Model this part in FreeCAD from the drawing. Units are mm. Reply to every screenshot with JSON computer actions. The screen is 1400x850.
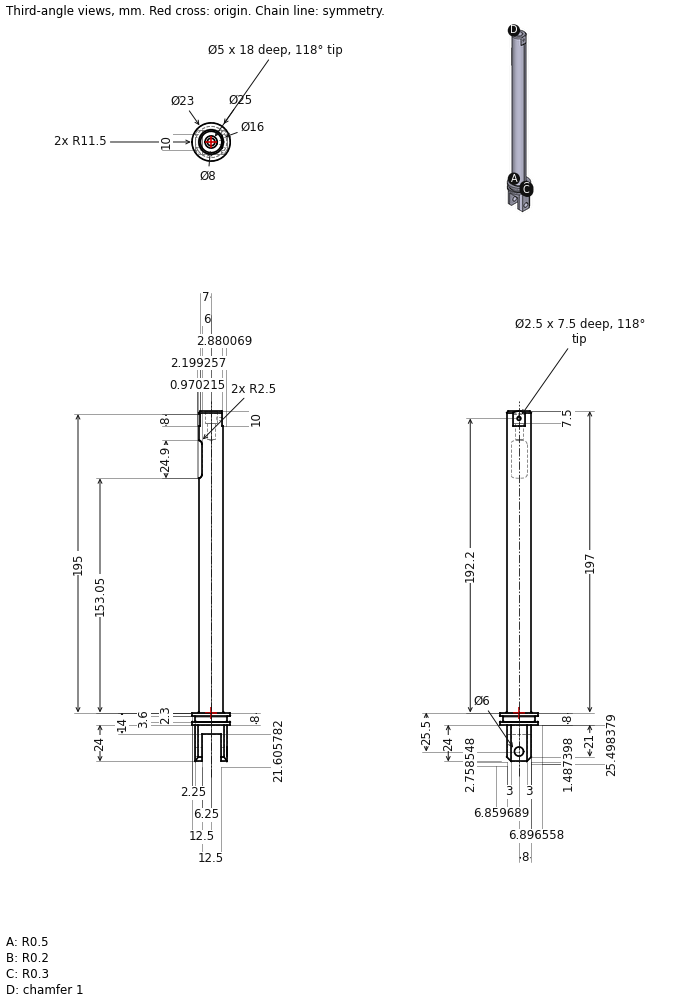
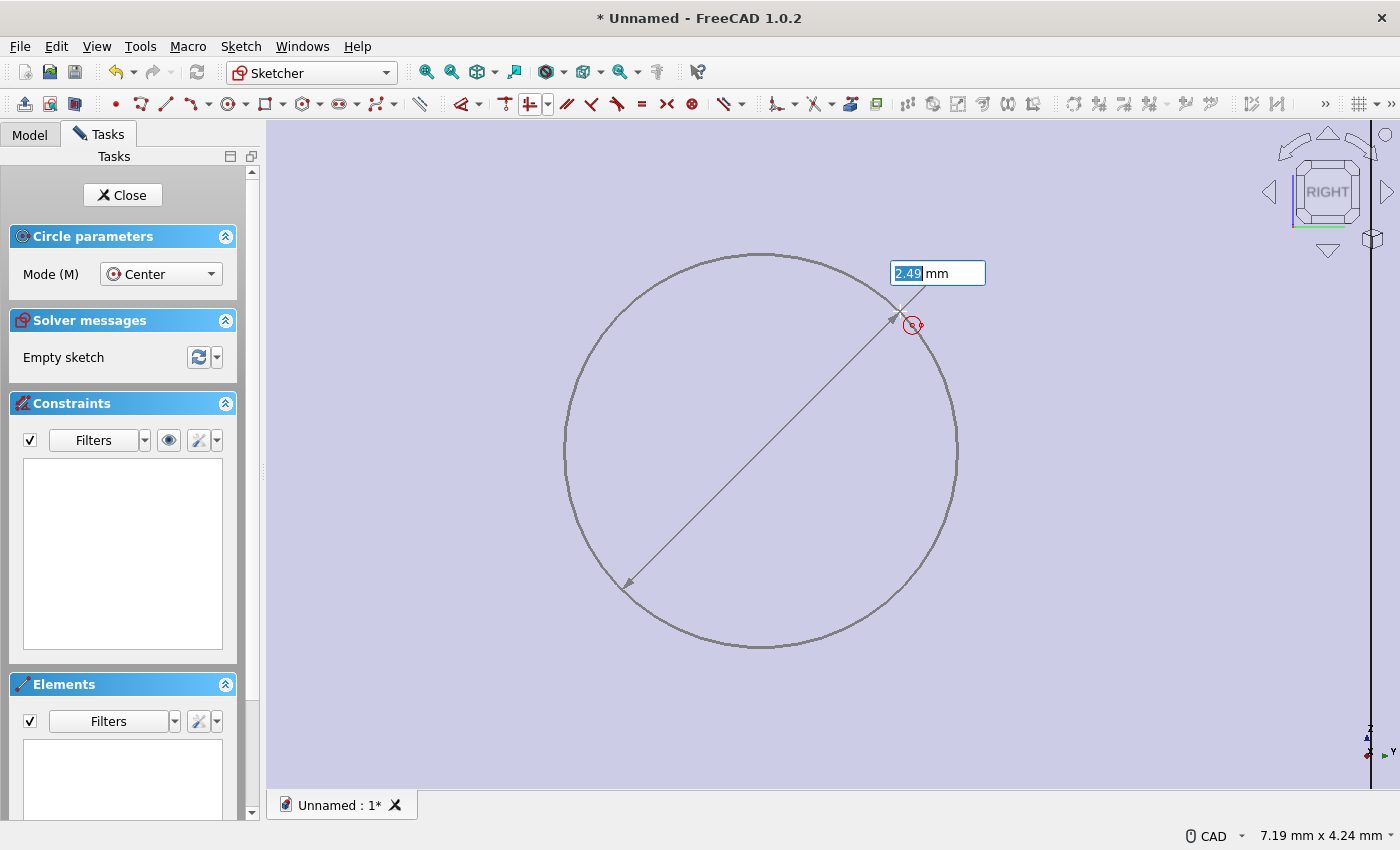
{"action": "type", "text": "2.5"}
{"action": "key", "text": "Return"}
{"action": "key", "text": "Escape"}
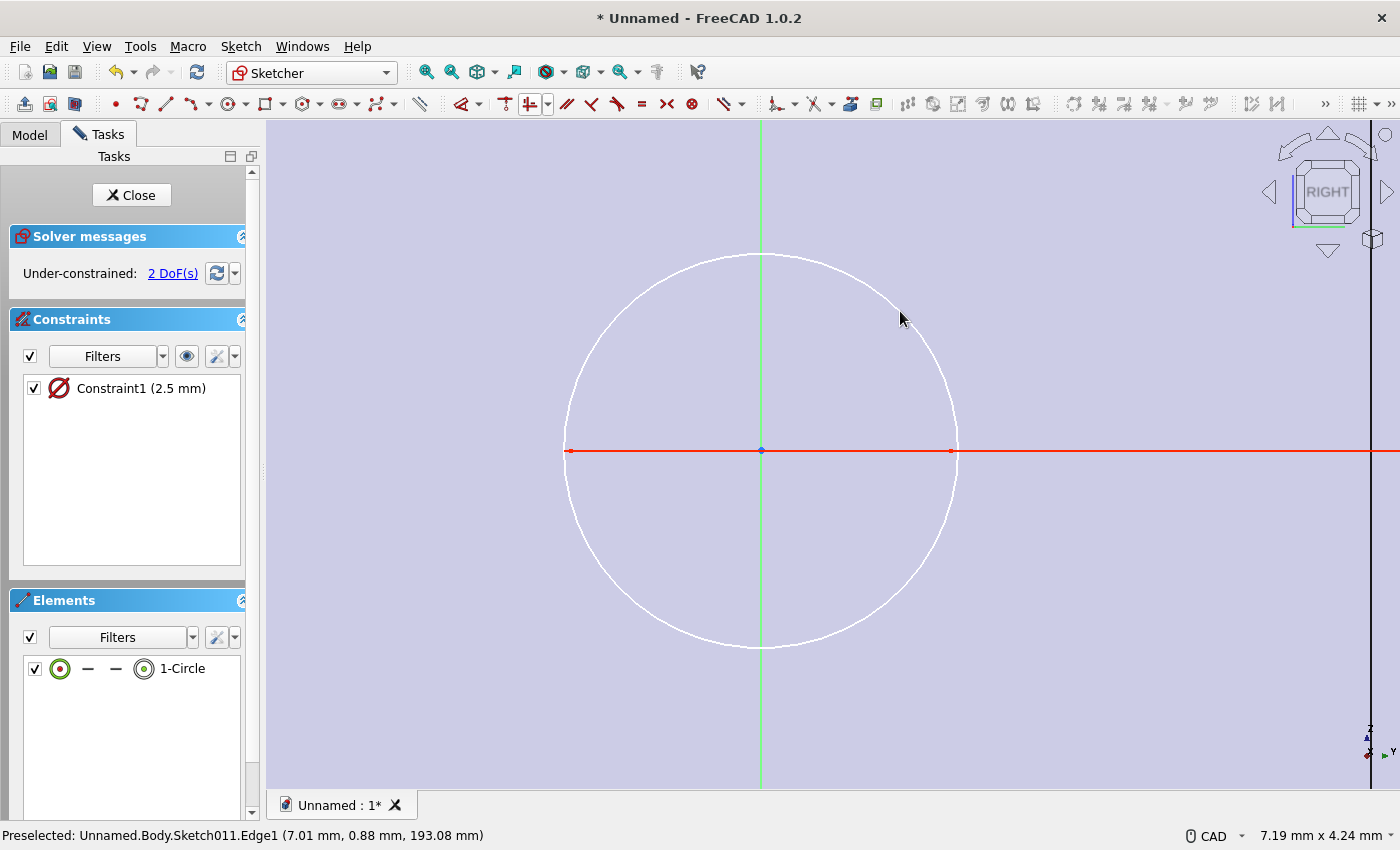
{"action": "left_click", "coordinate": [761, 451]}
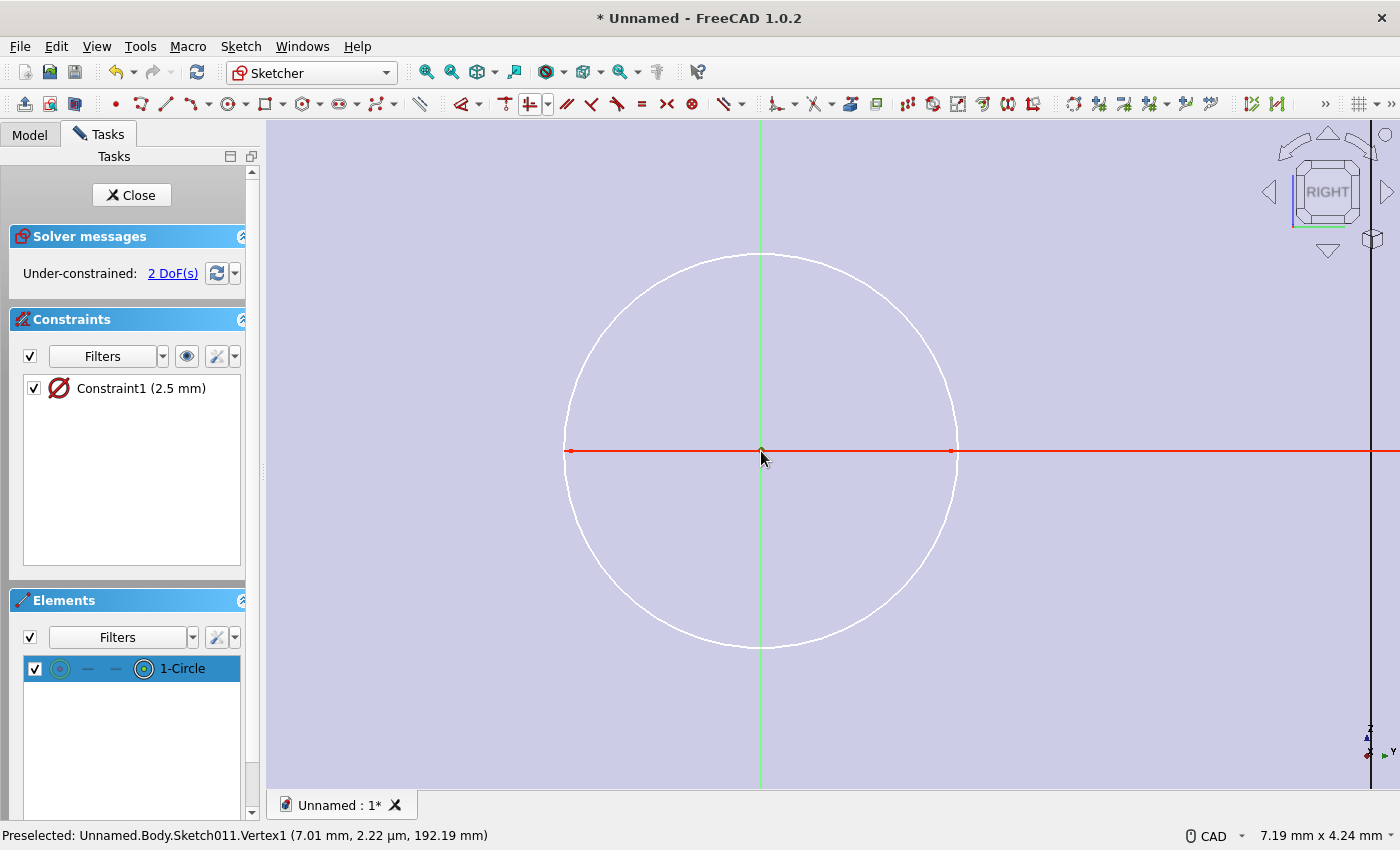
{"action": "left_click", "coordinate": [761, 717]}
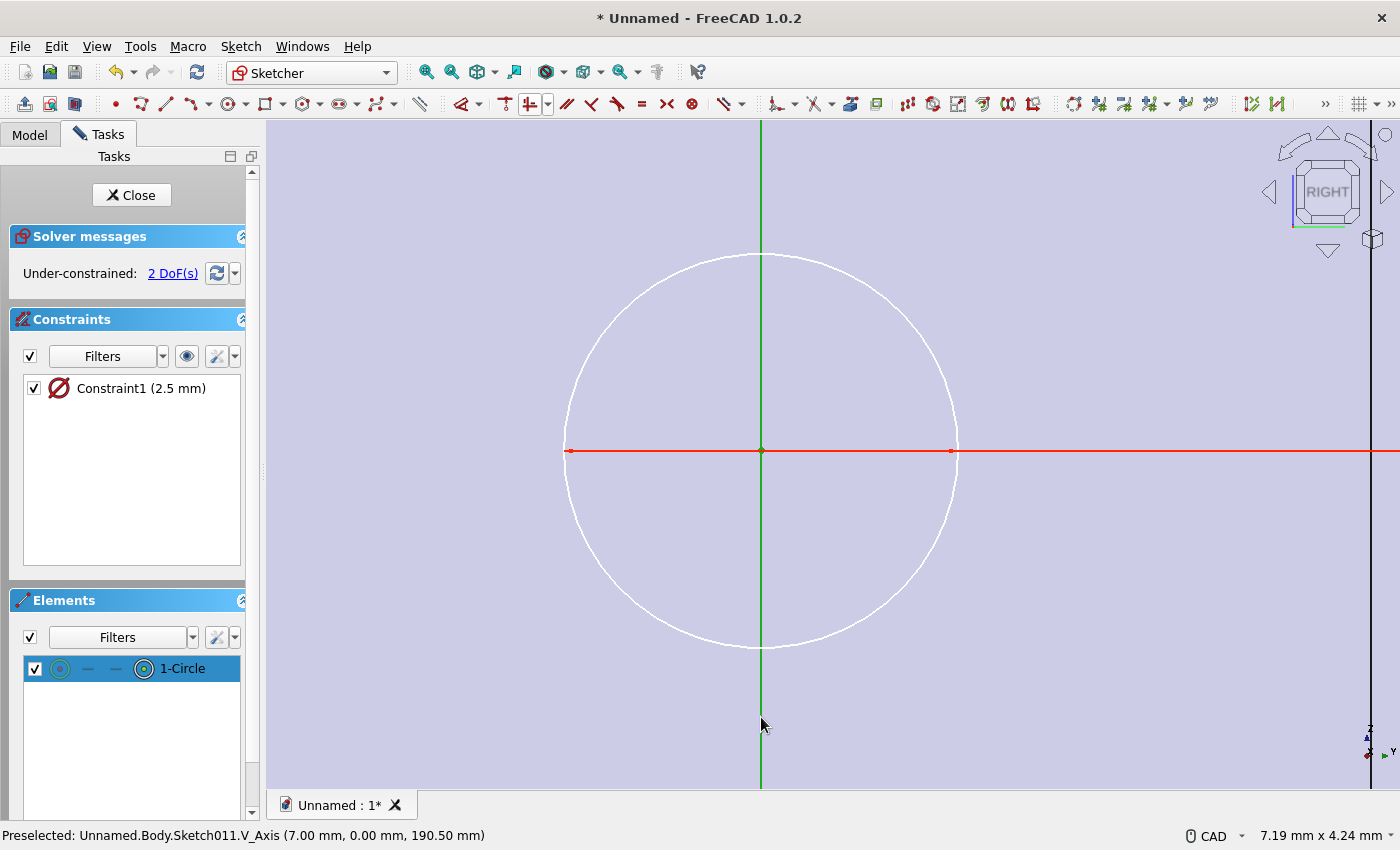
{"action": "left_click", "coordinate": [505, 104]}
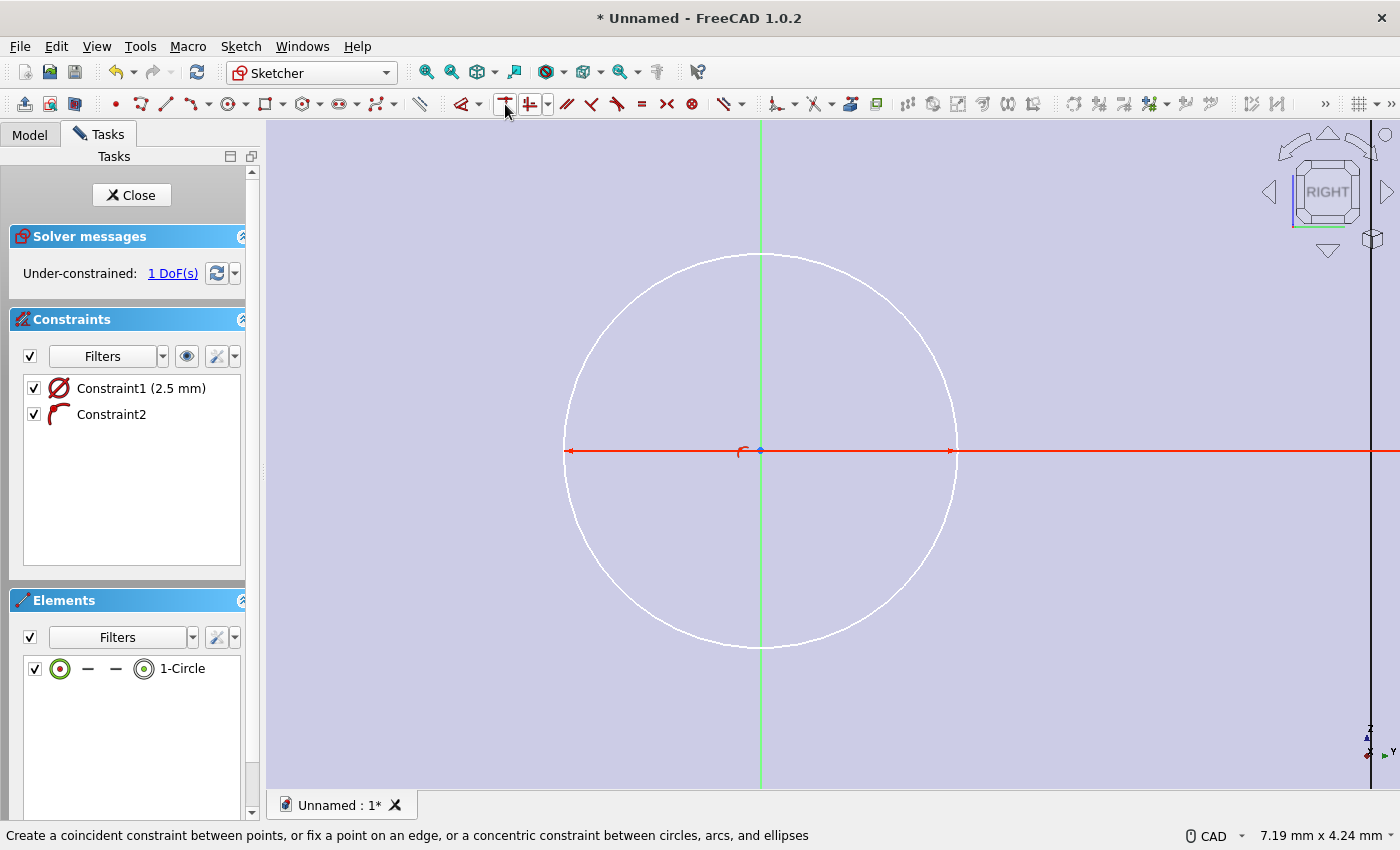
{"action": "left_click", "coordinate": [460, 104]}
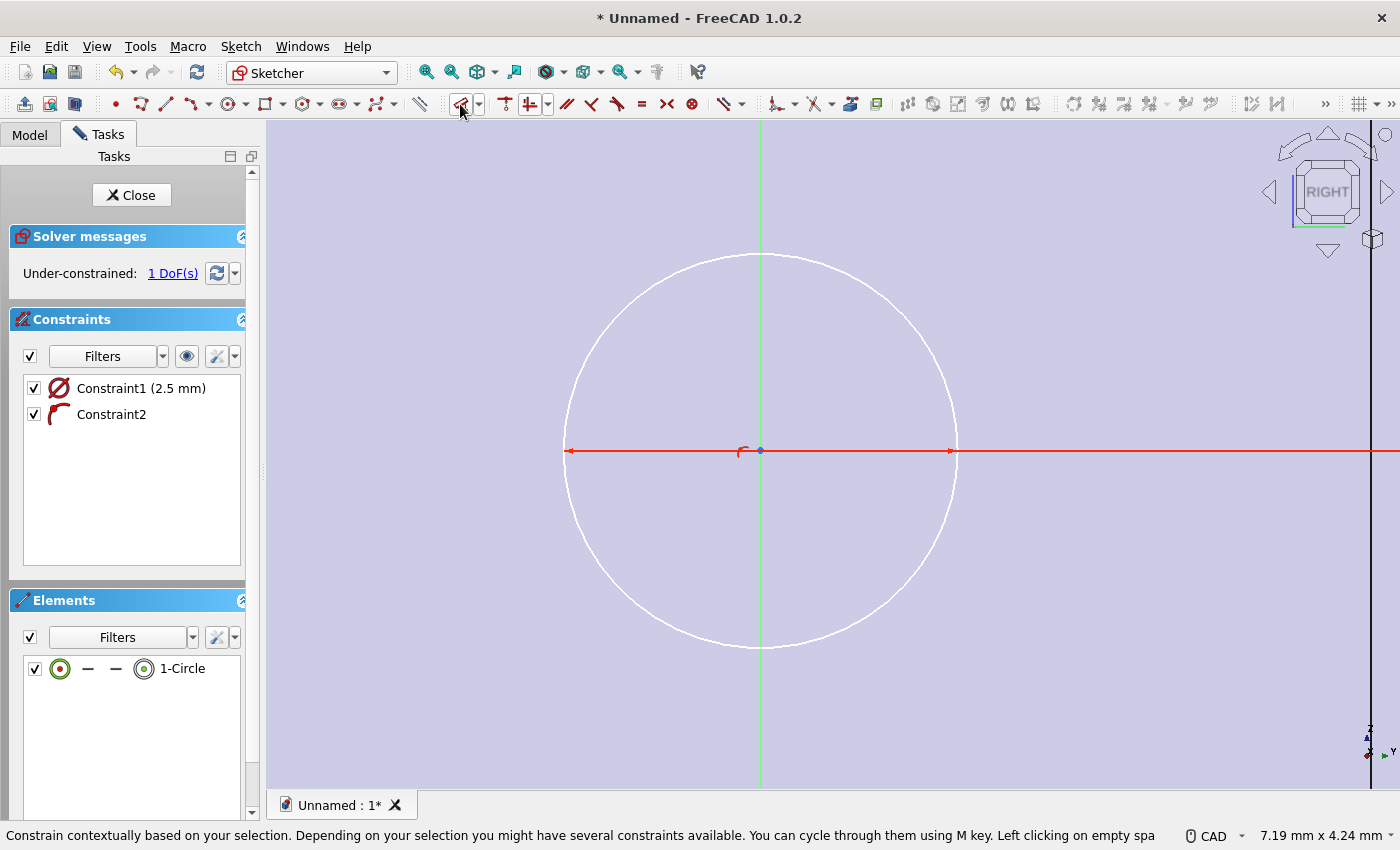
{"action": "left_click", "coordinate": [761, 451]}
{"action": "left_click", "coordinate": [795, 606]}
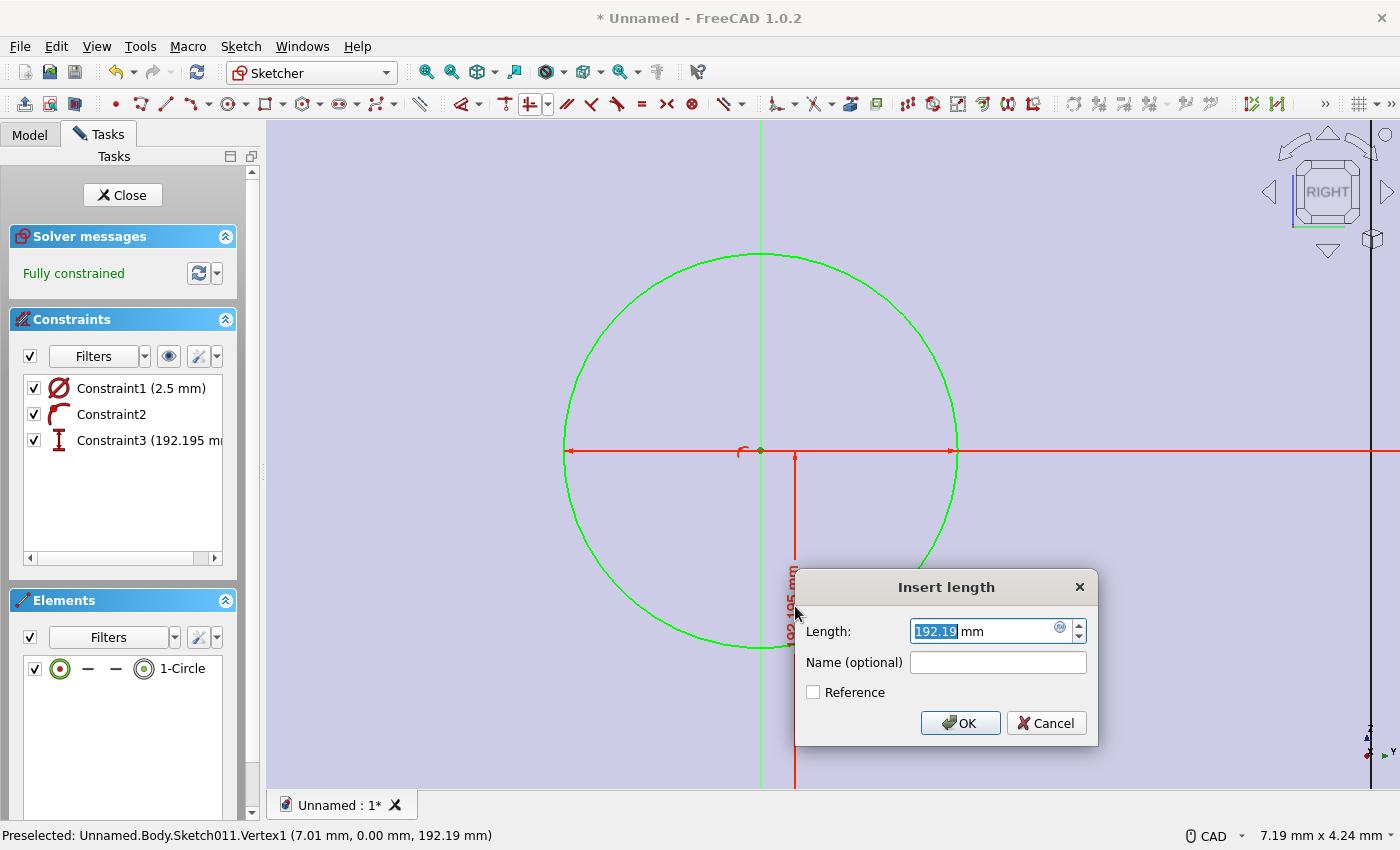
{"action": "type", "text": "192.2"}
{"action": "key", "text": "Return"}
{"action": "key", "text": "Escape"}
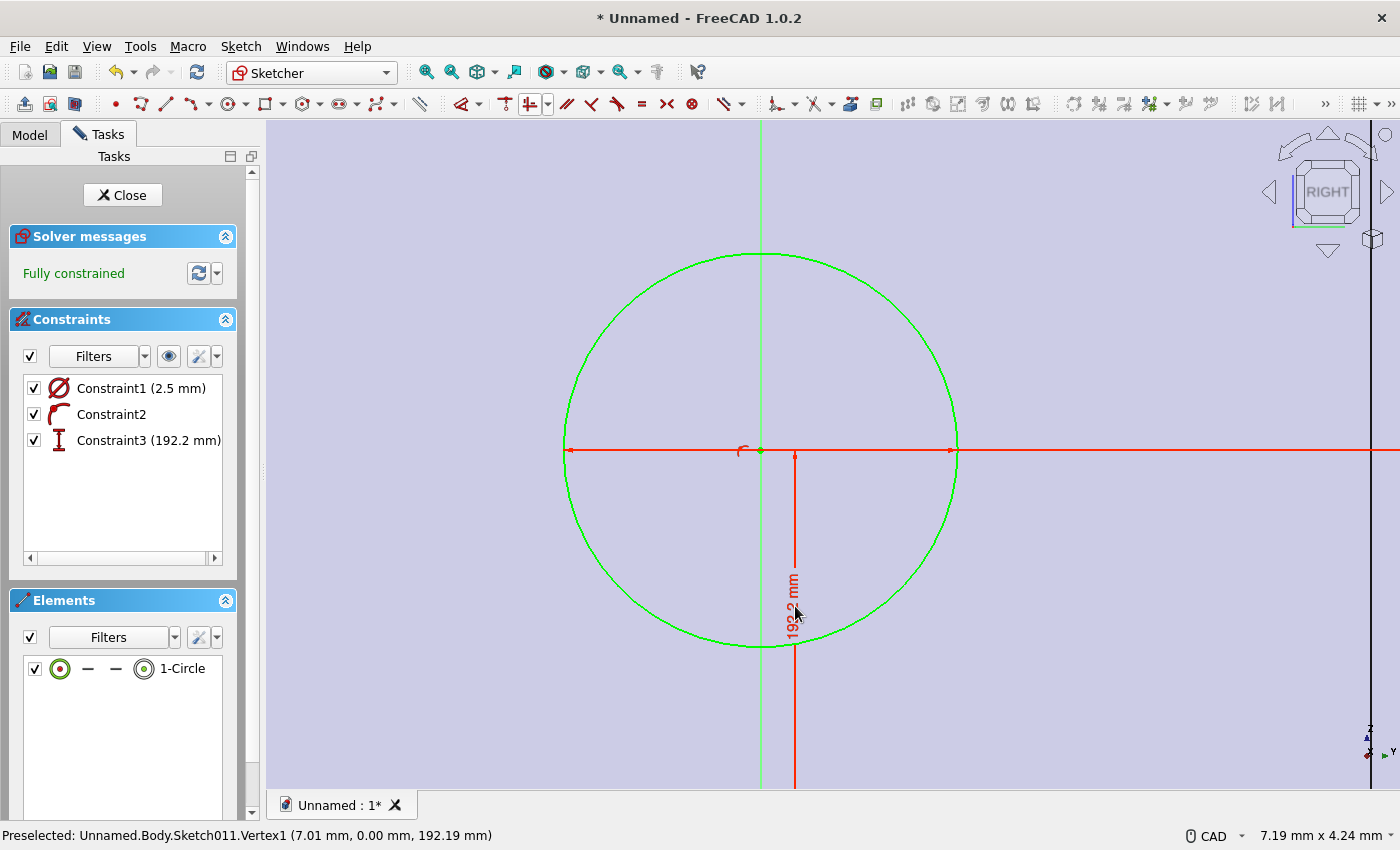
{"action": "left_click", "coordinate": [123, 195]}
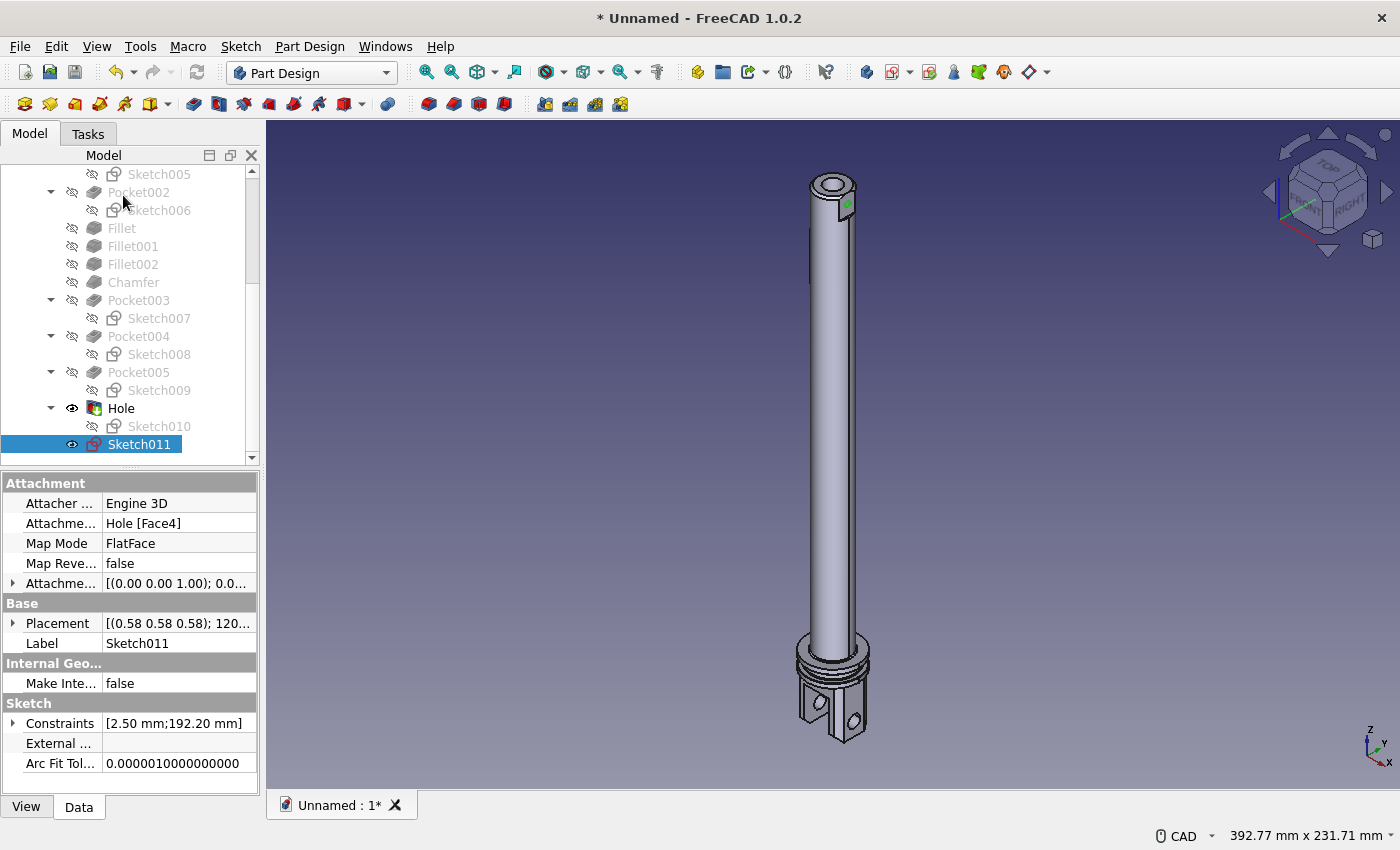
{"action": "left_click", "coordinate": [219, 104]}